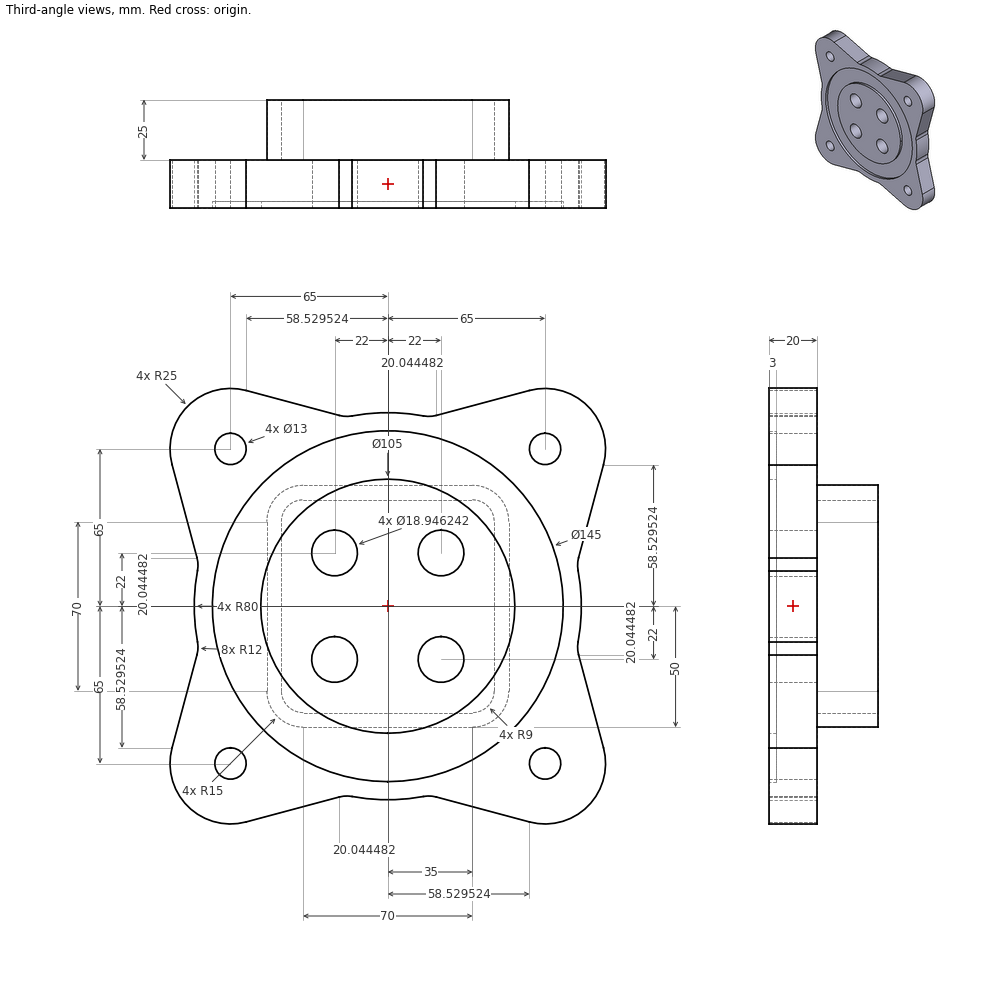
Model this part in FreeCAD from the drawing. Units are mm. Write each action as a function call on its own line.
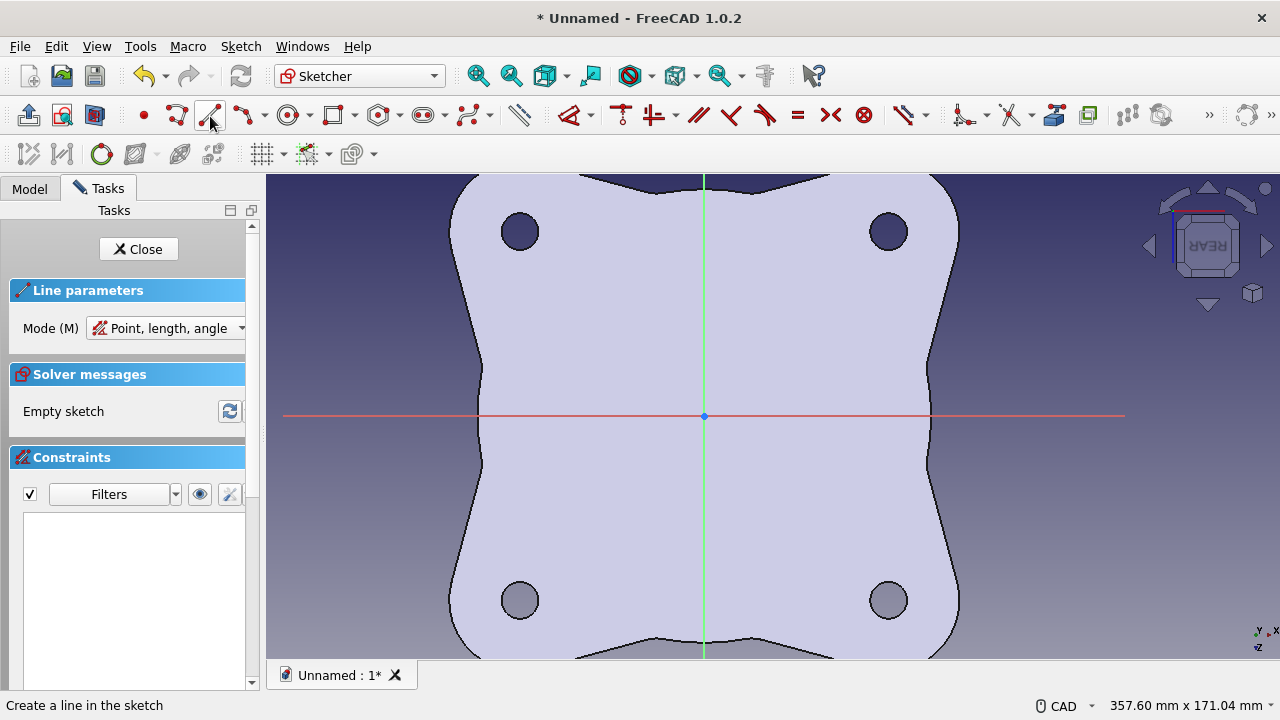
click(804, 274)
click(605, 274)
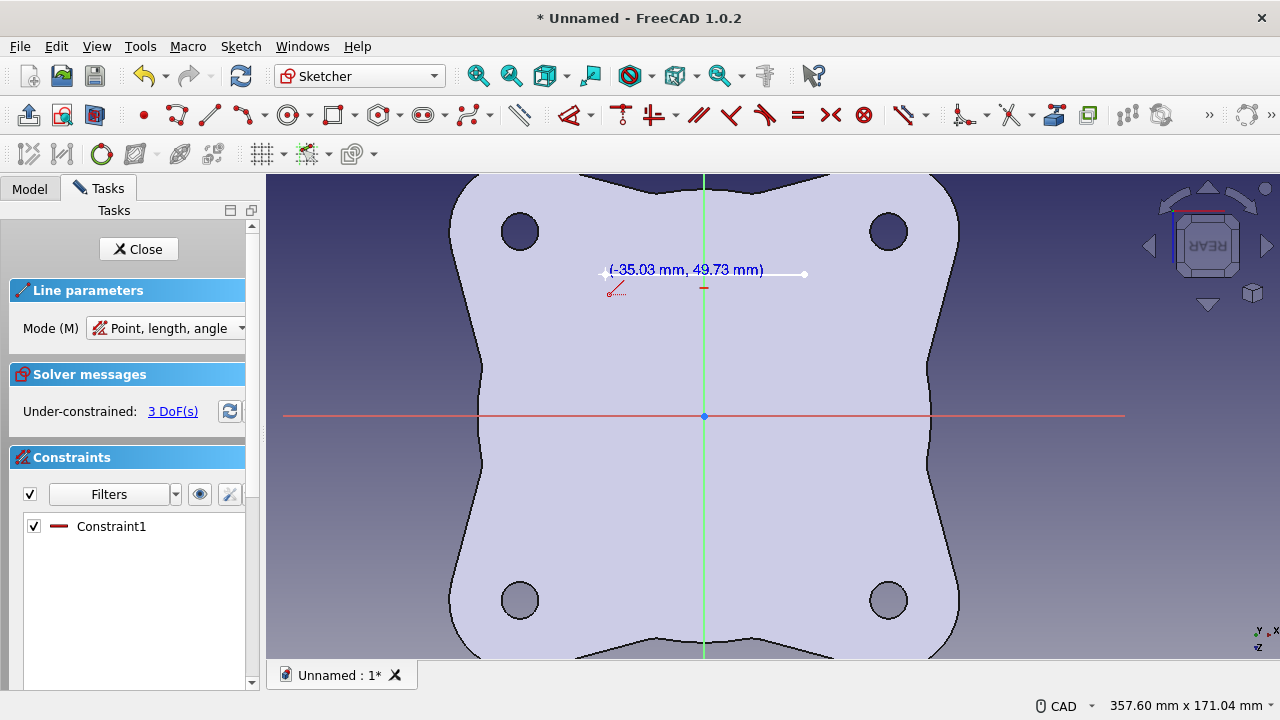
click(563, 317)
click(563, 515)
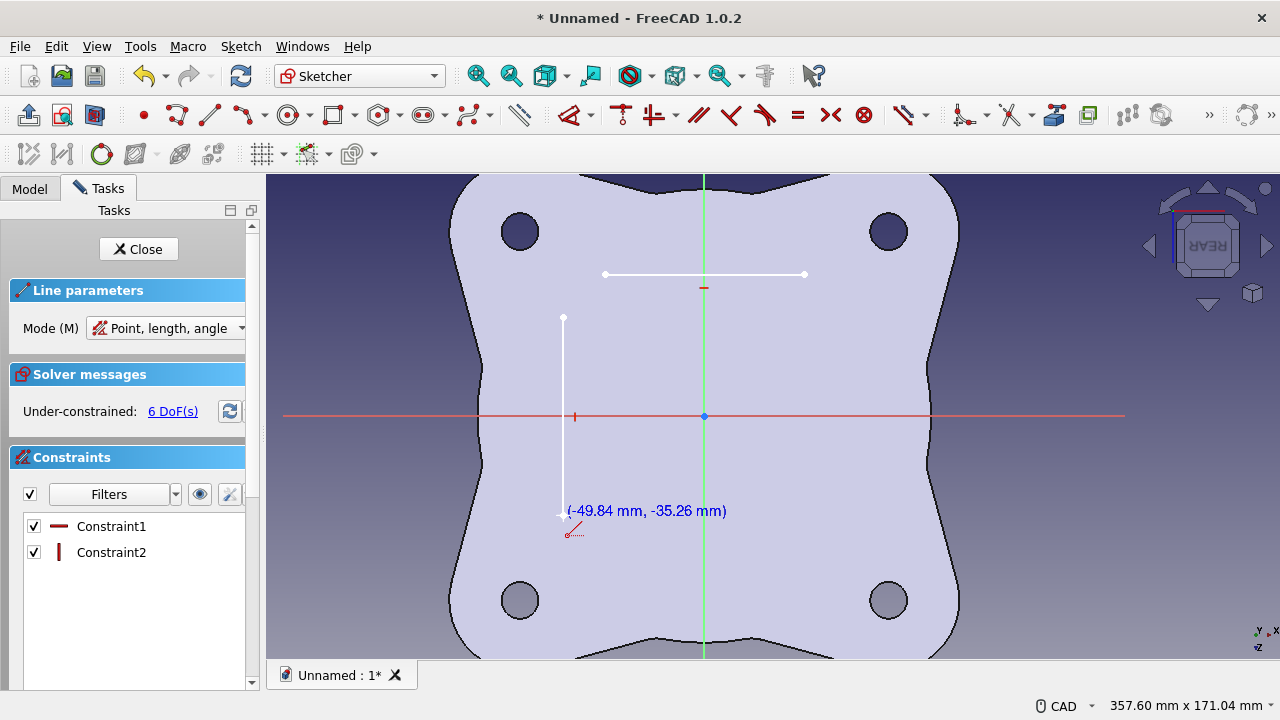
click(605, 558)
click(804, 558)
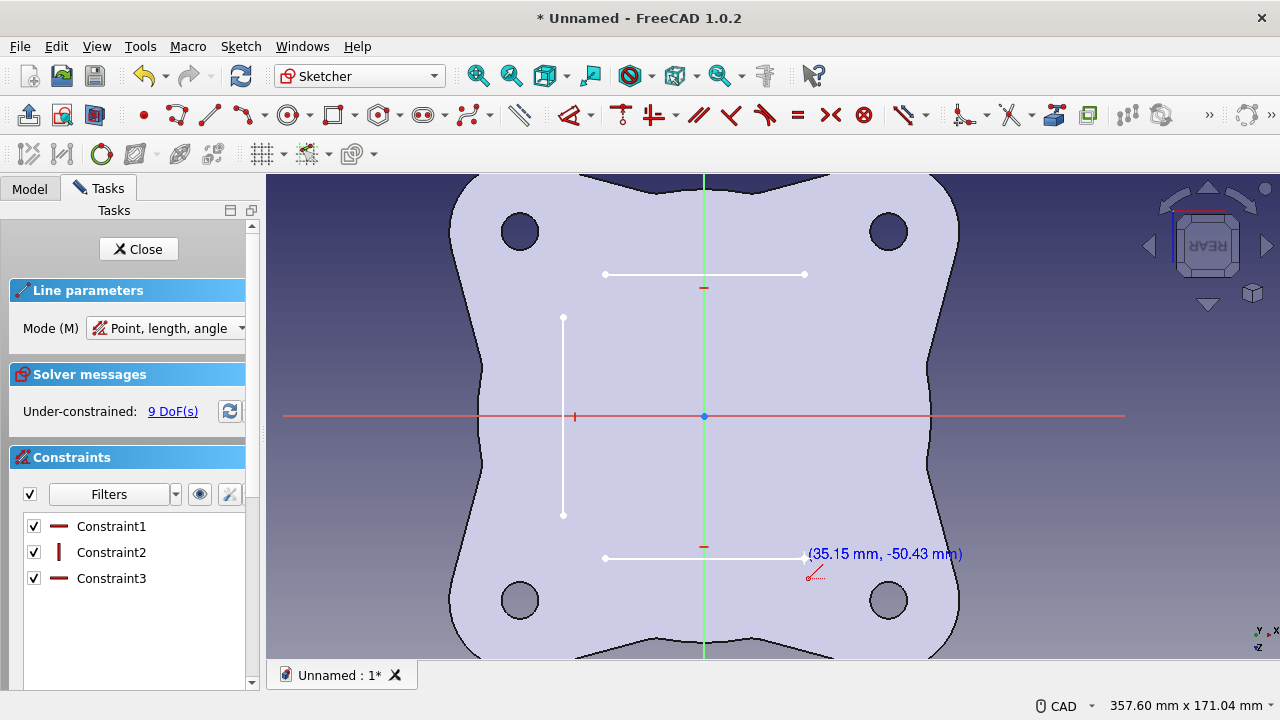
click(846, 515)
click(846, 317)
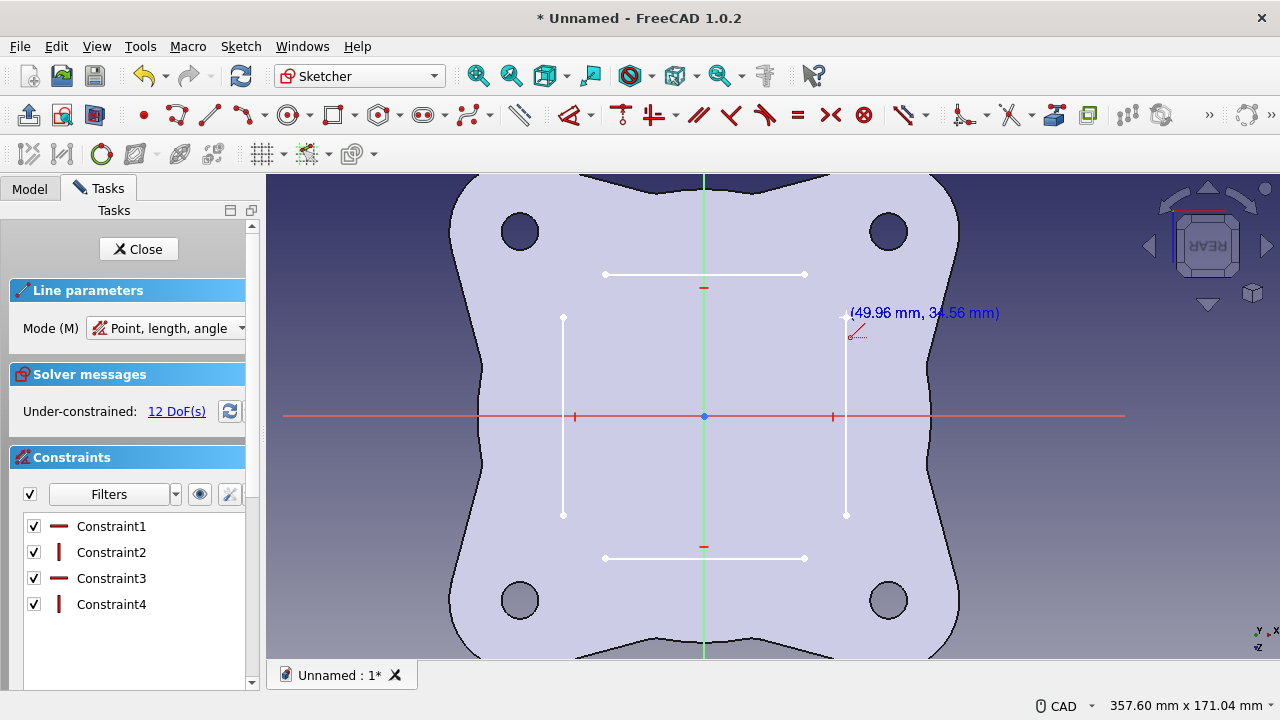
click(242, 116)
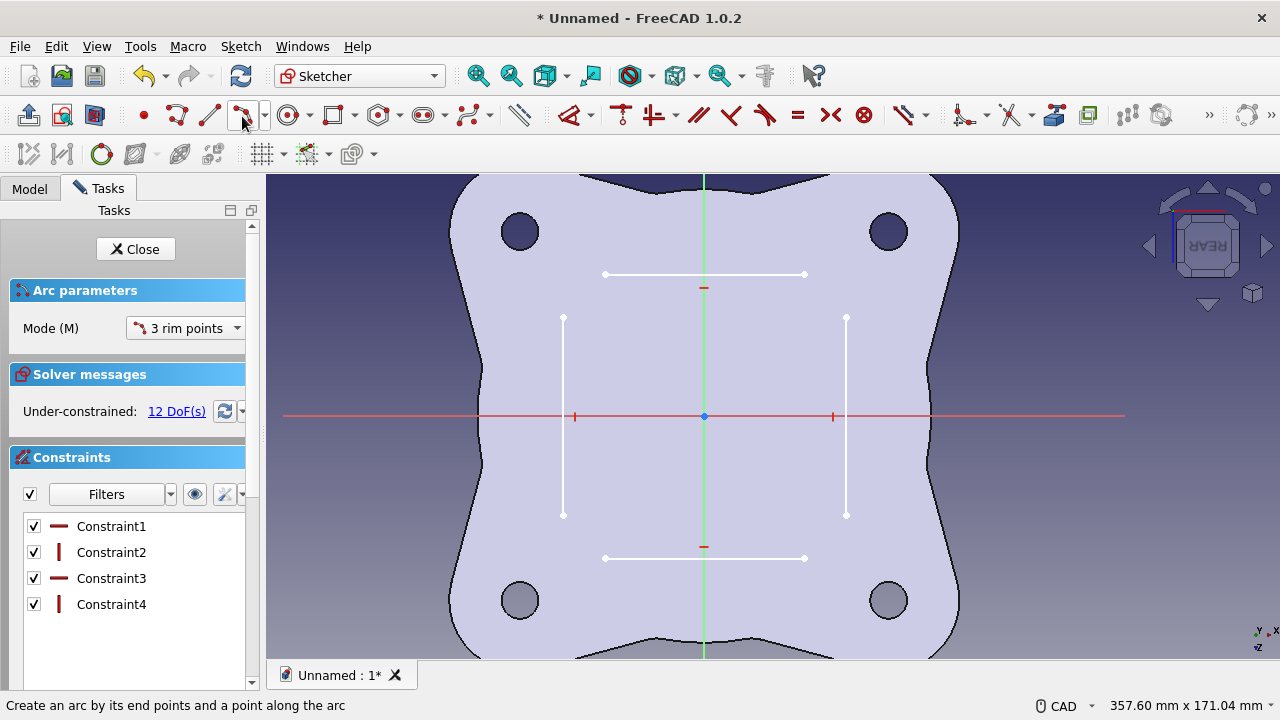
click(605, 275)
click(563, 318)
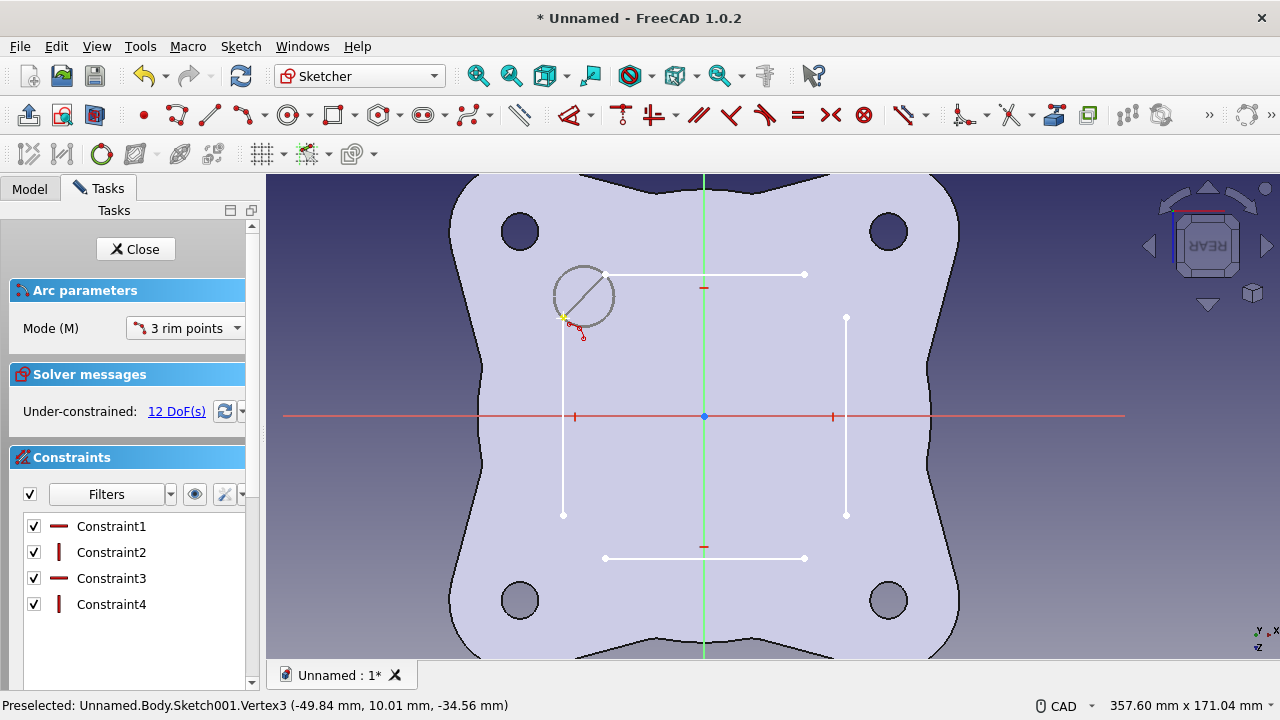
scroll(575, 287, up, 2)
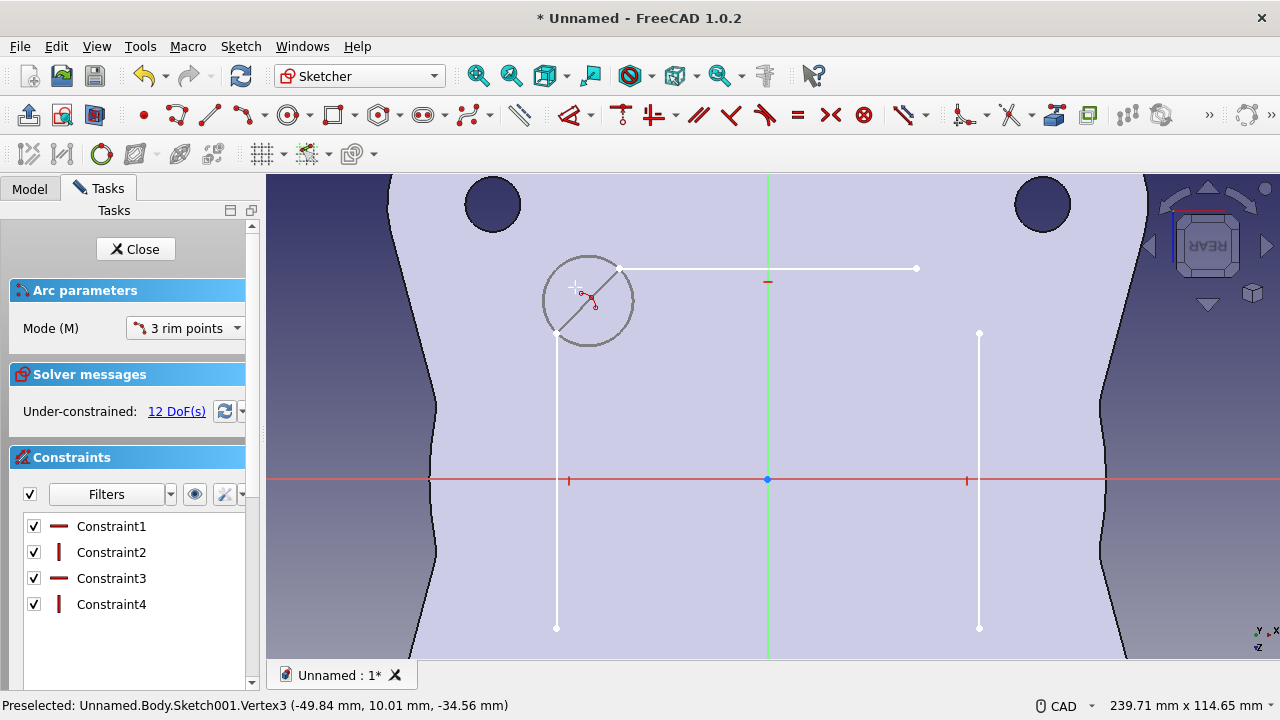
click(575, 286)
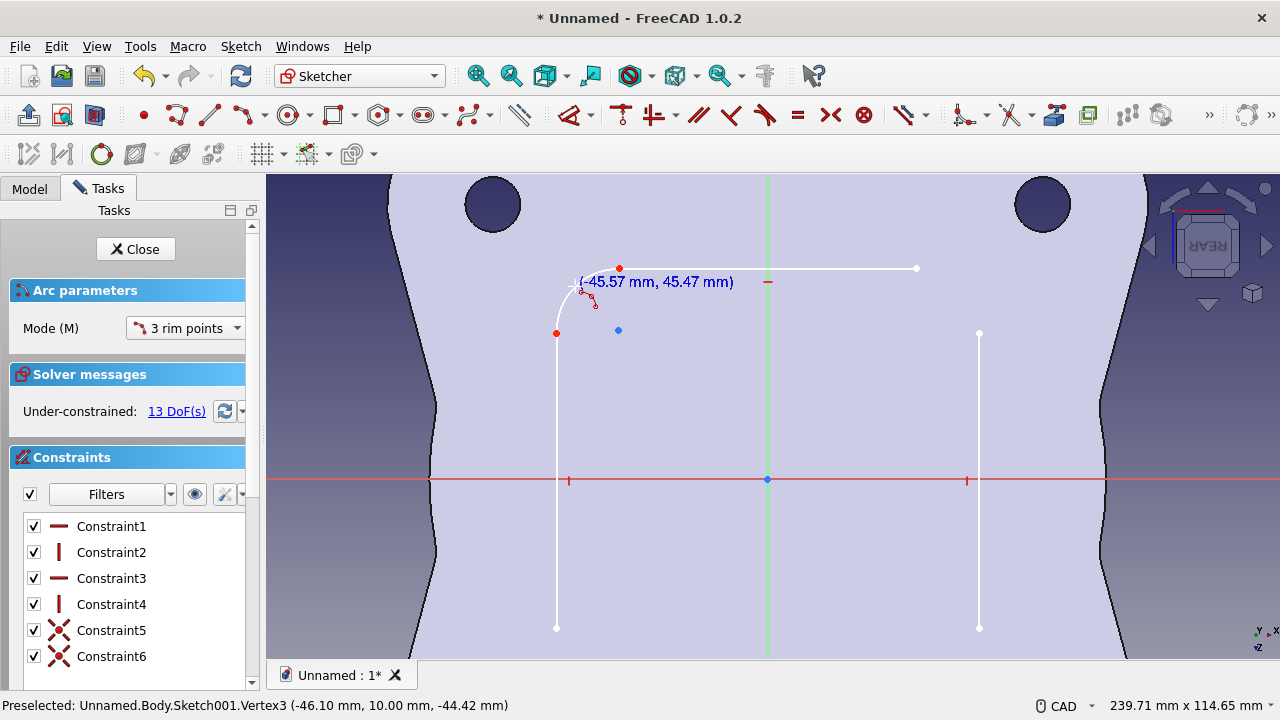
click(557, 629)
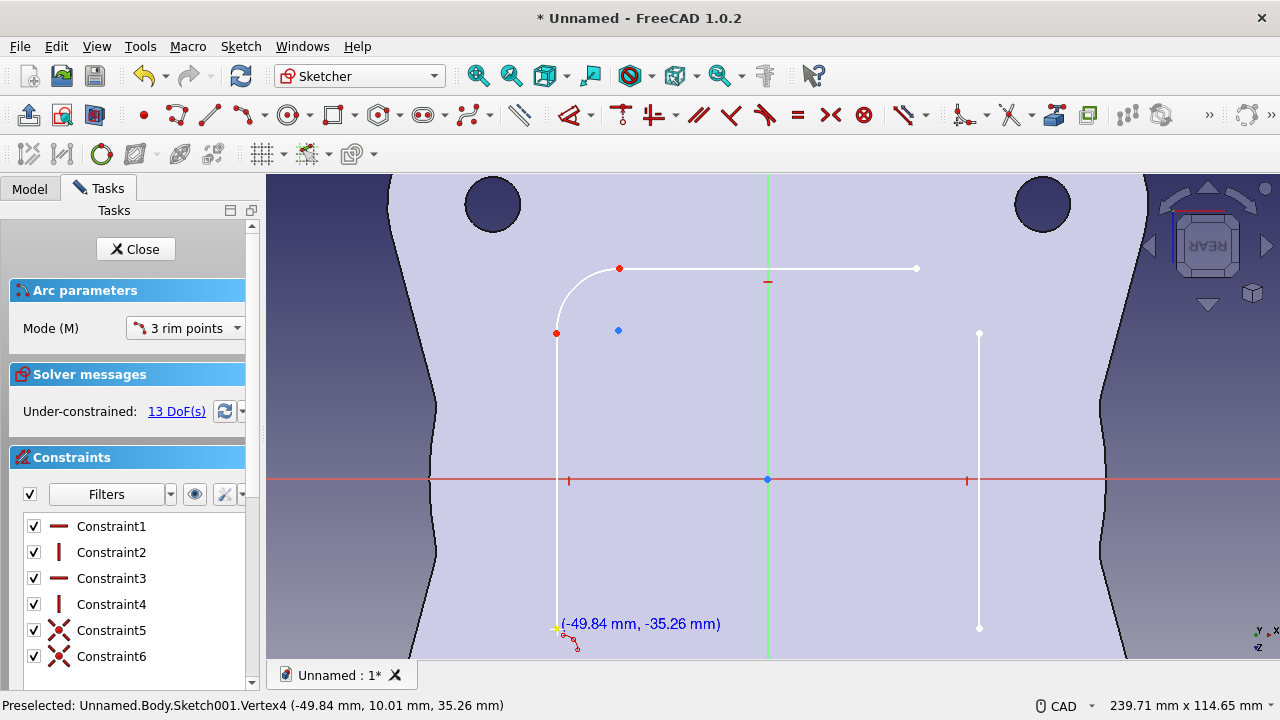
scroll(576, 289, down, 2)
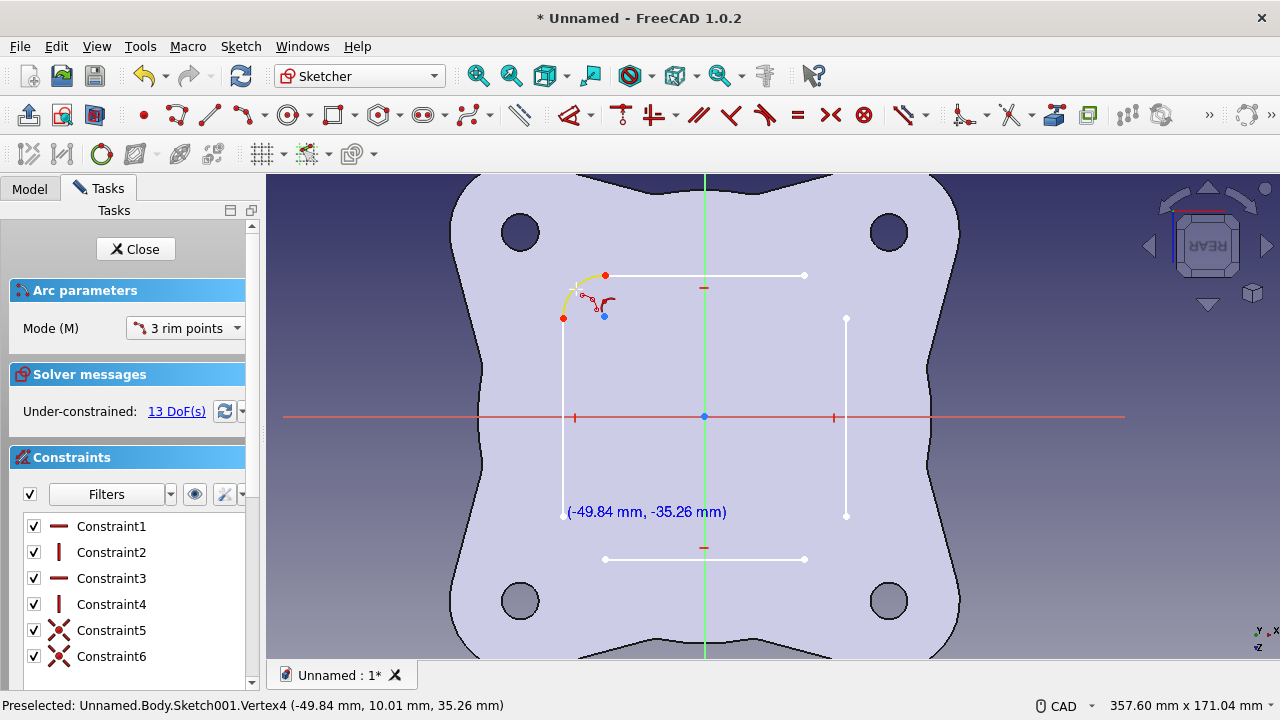
click(605, 560)